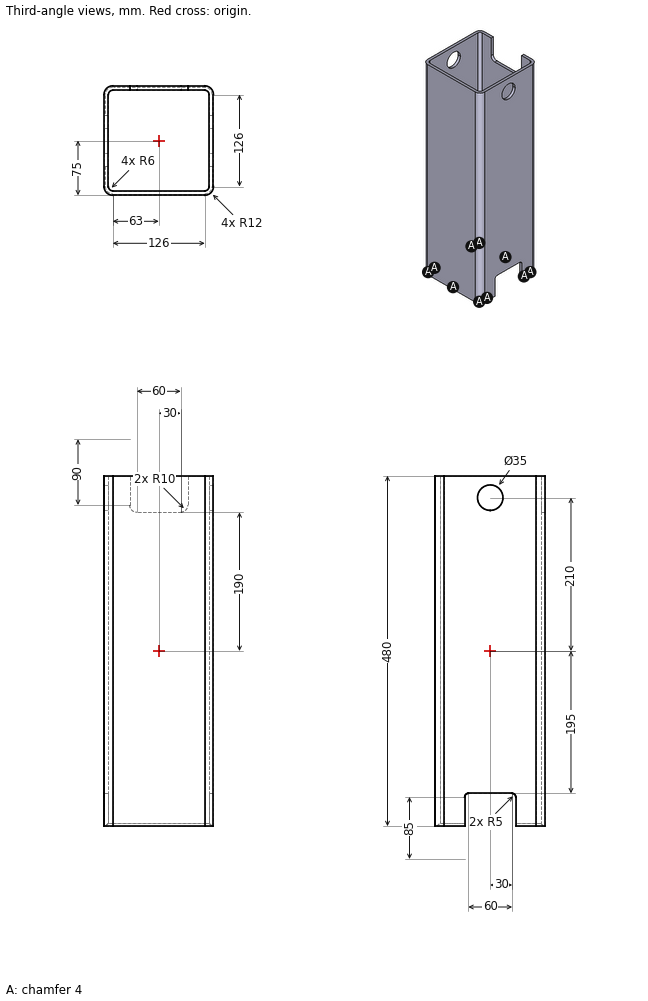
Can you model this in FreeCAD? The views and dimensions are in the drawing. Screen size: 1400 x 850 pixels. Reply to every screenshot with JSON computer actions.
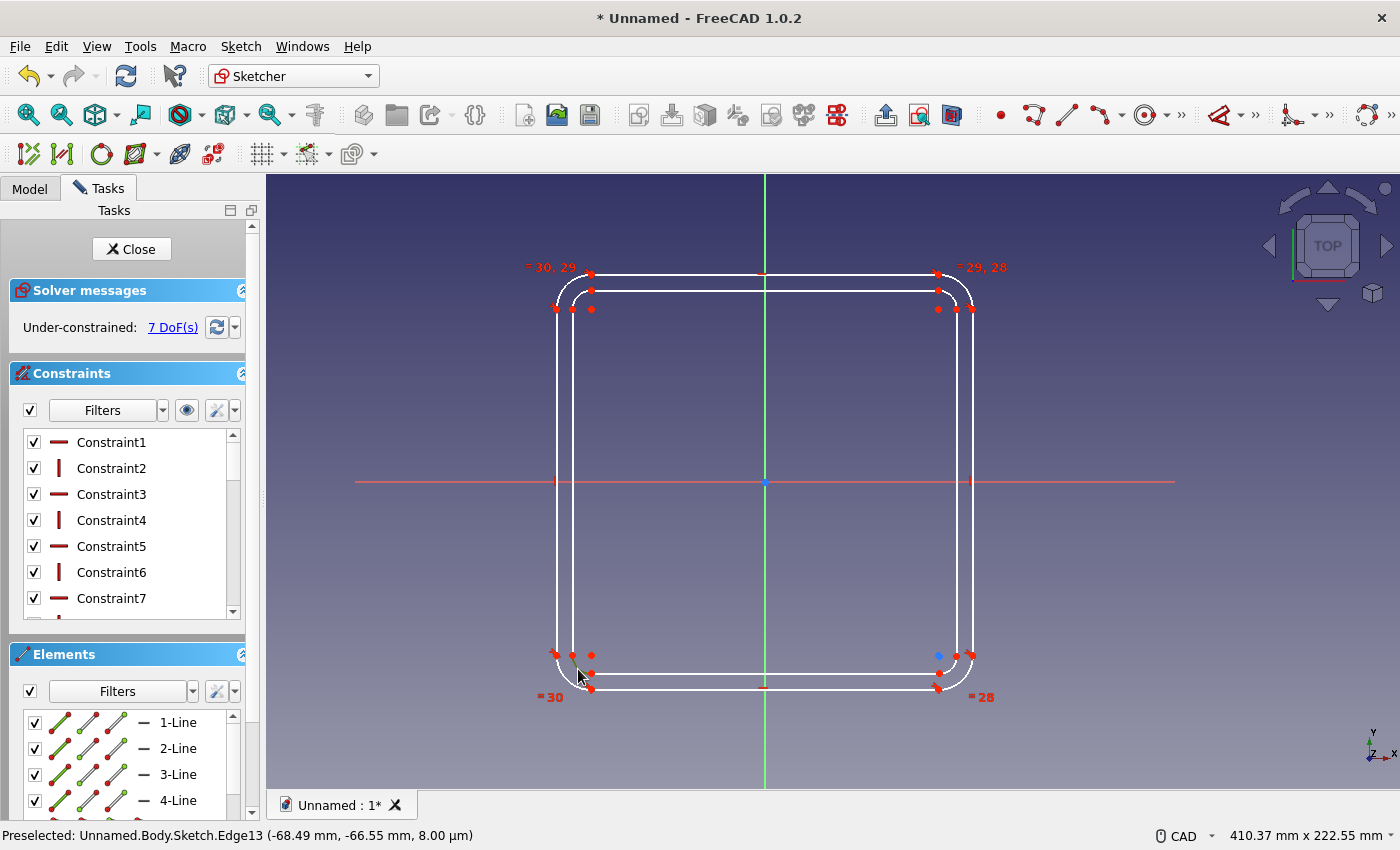
{"action": "left_click", "coordinate": [952, 669]}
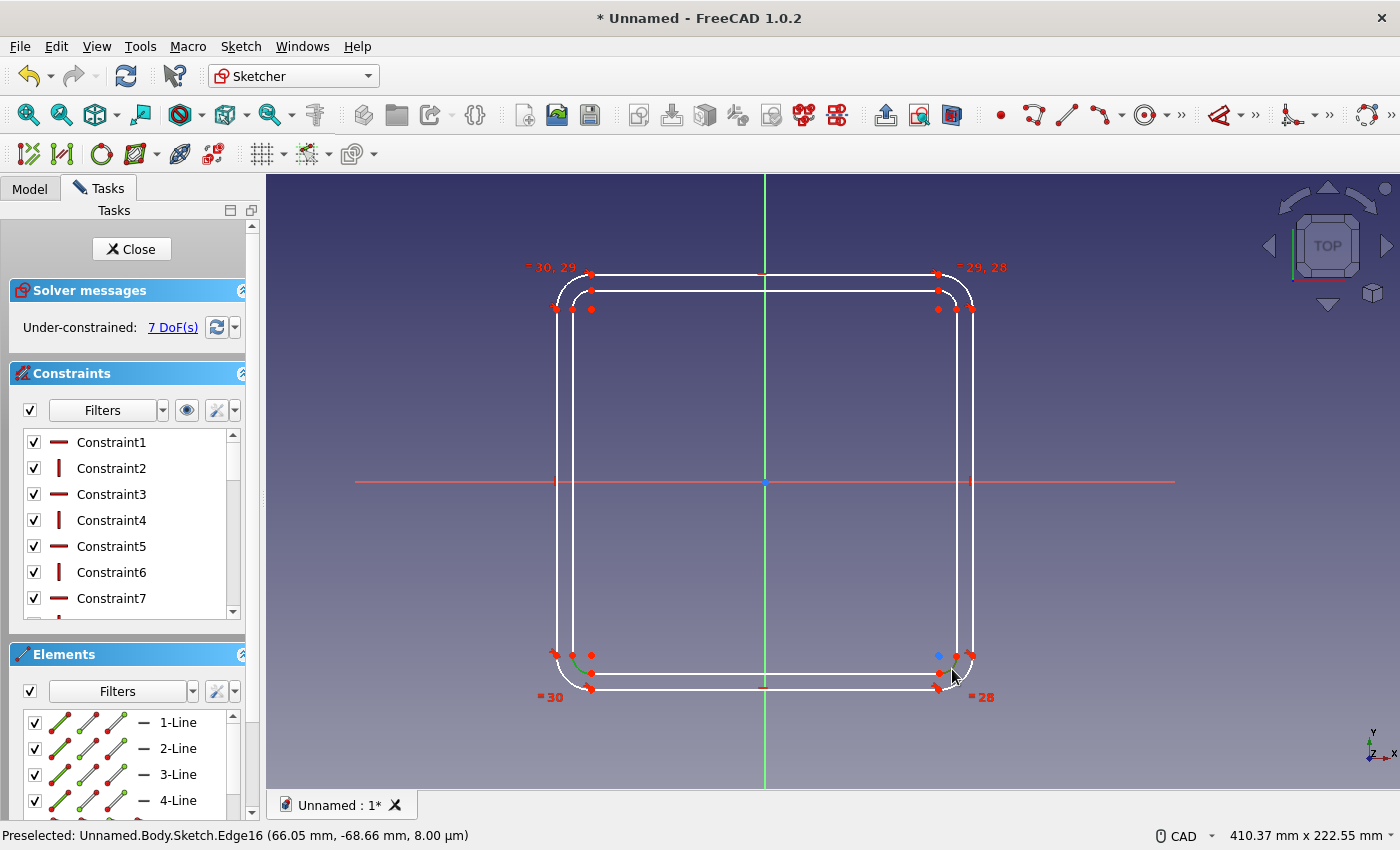
{"action": "key", "text": "e"}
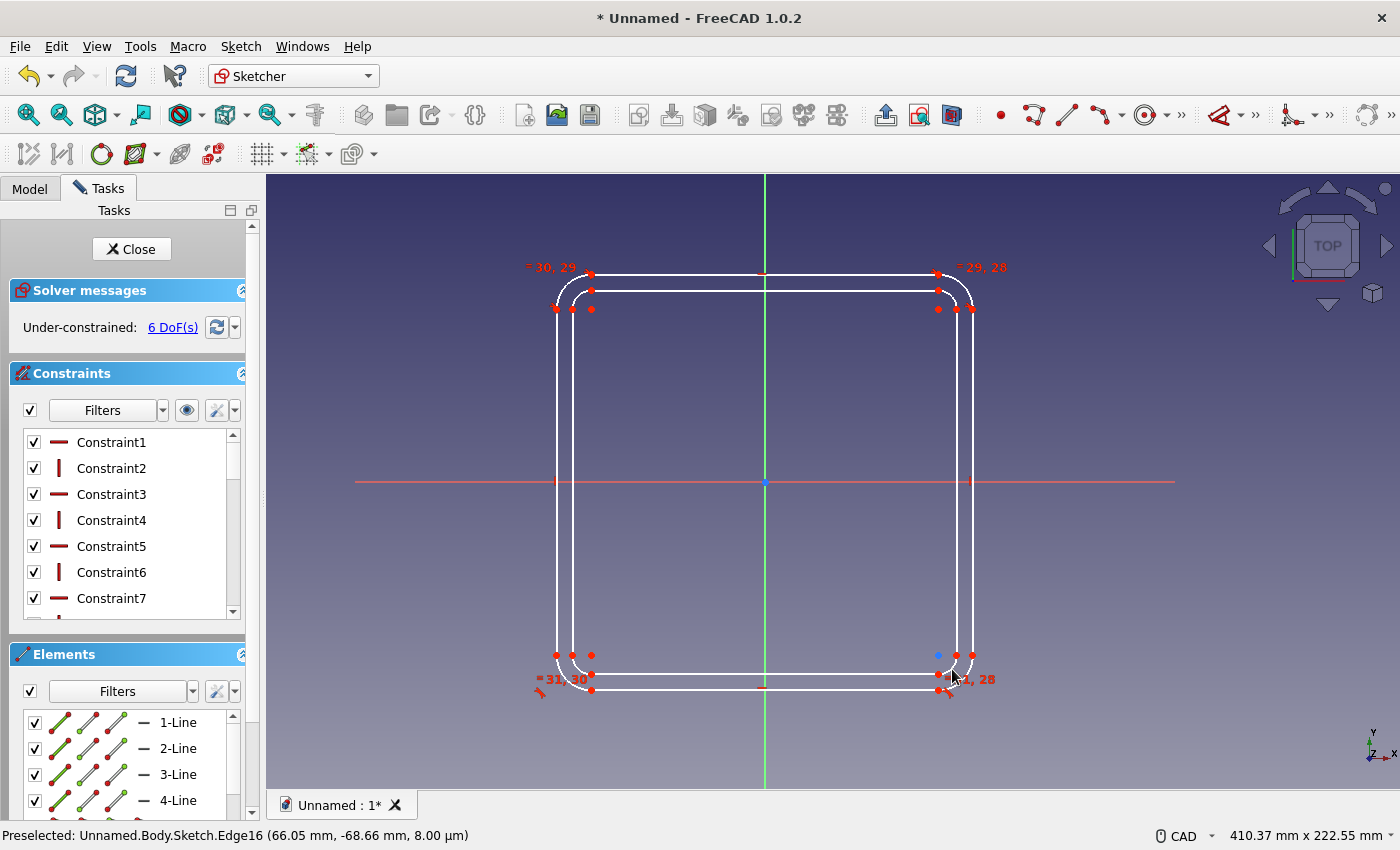
{"action": "left_click", "coordinate": [971, 667]}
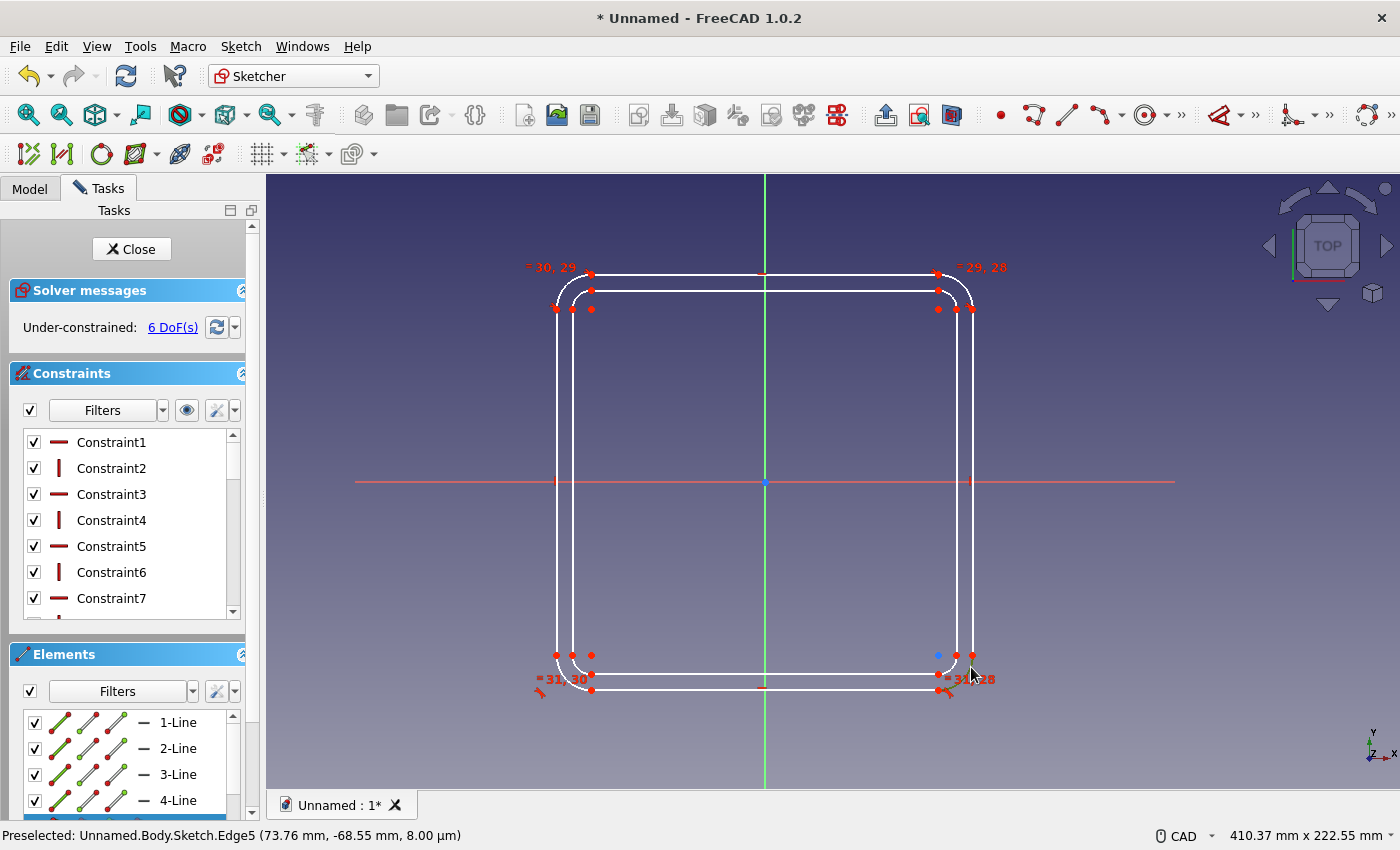
{"action": "key", "text": "k r"}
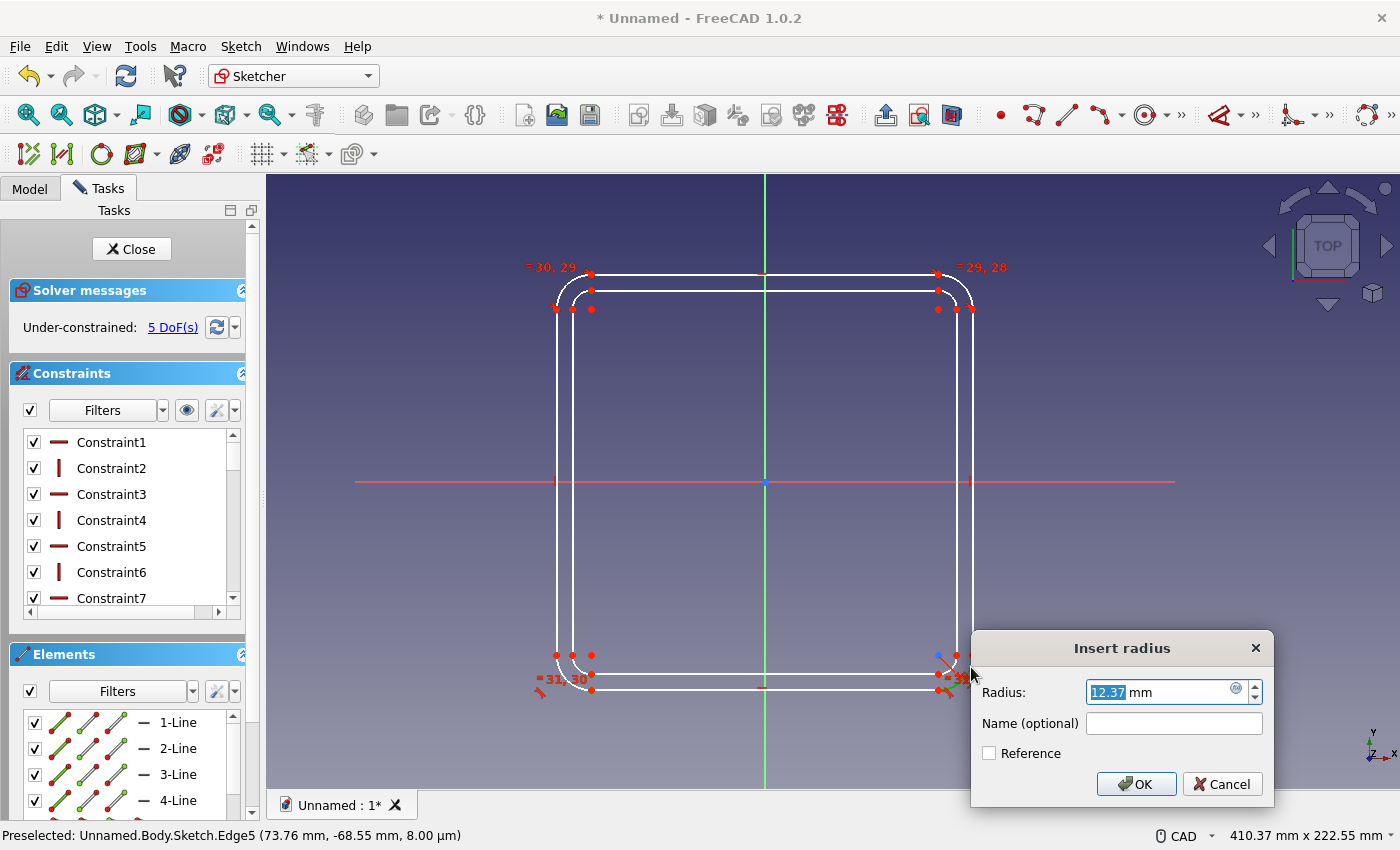
{"action": "type", "text": "12"}
{"action": "key", "text": "Return"}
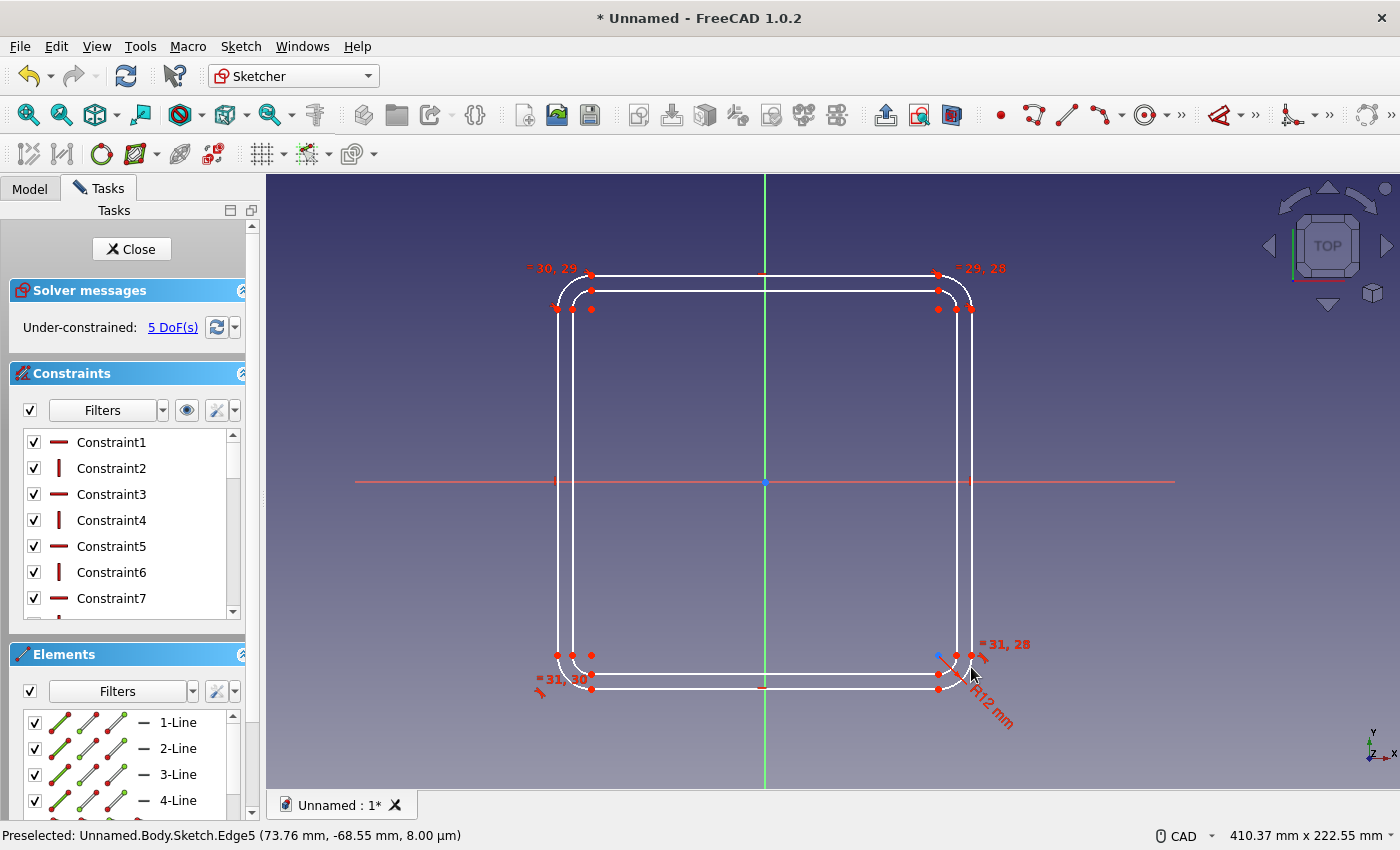
{"action": "scroll", "coordinate": [578, 669], "scroll_direction": "up", "scroll_amount": 5}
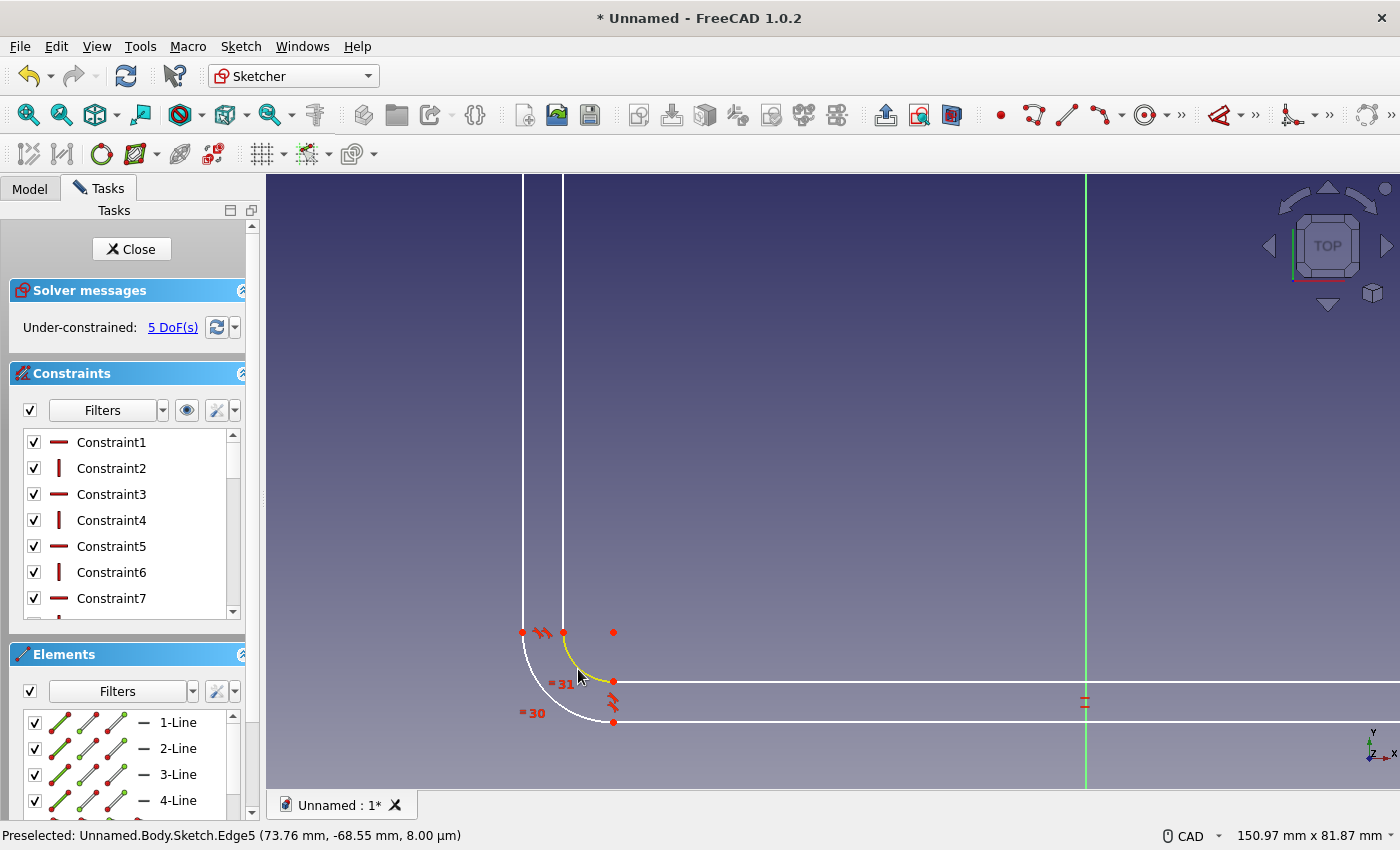
{"action": "left_click", "coordinate": [578, 667]}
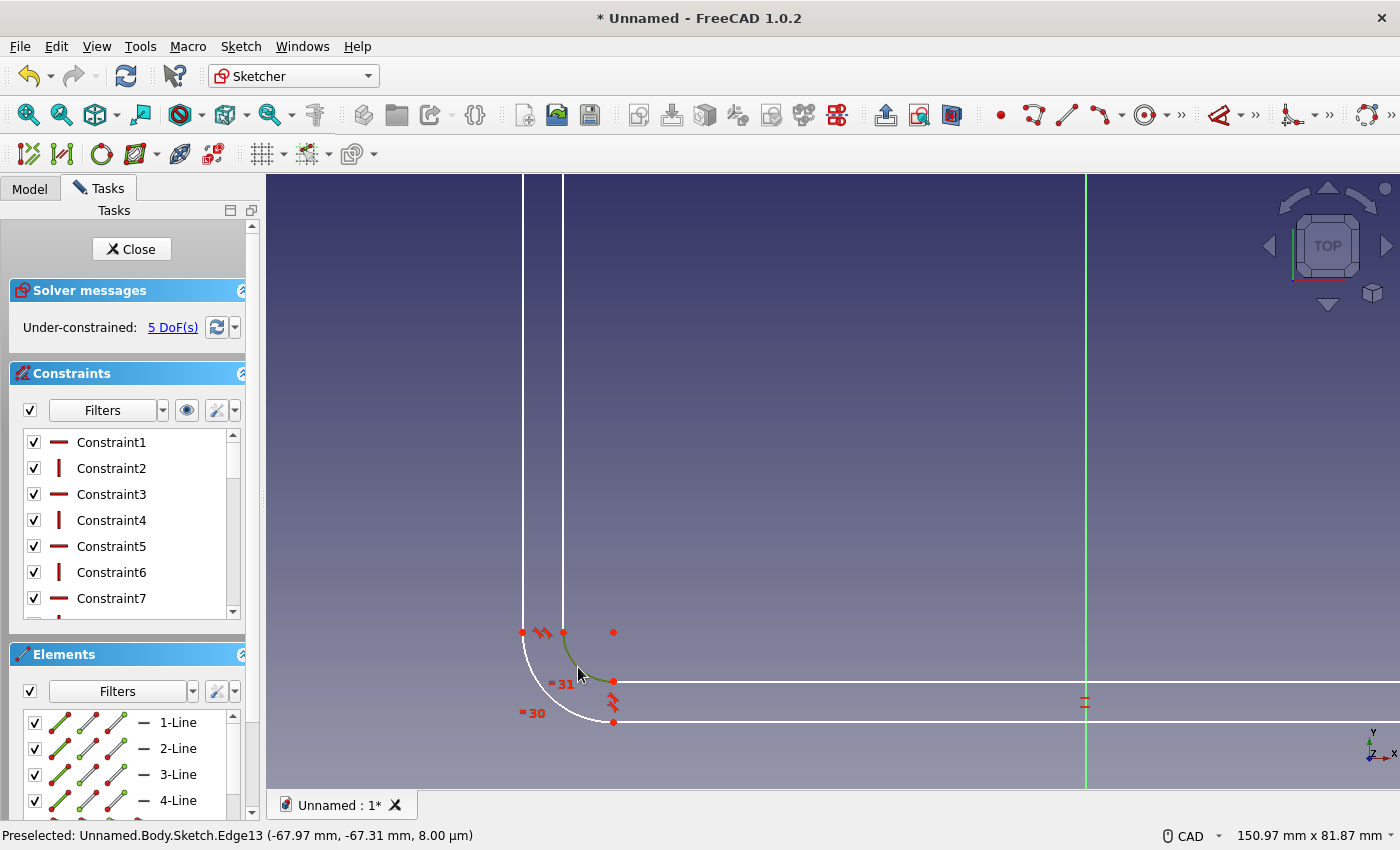
{"action": "key", "text": "k r"}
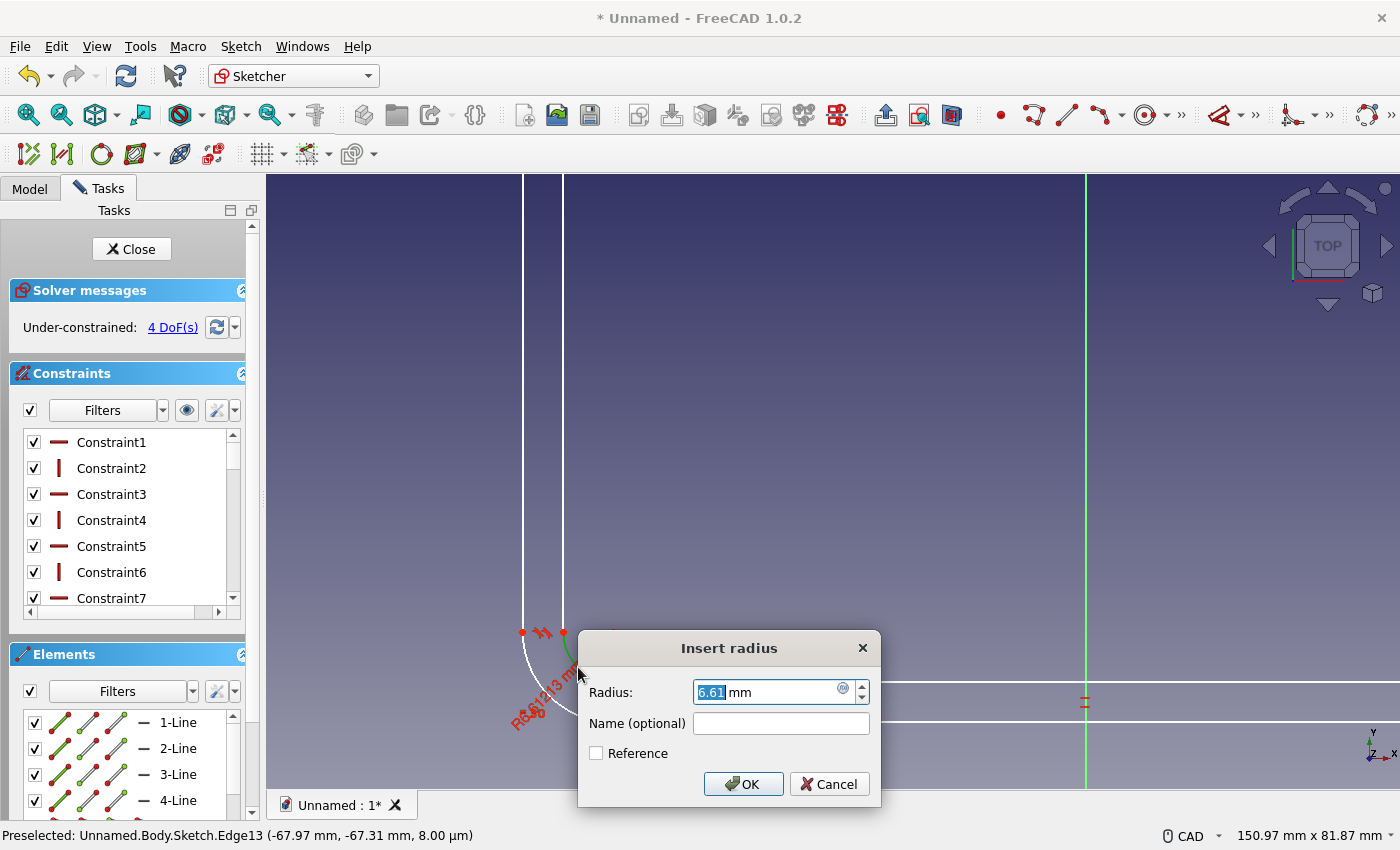
{"action": "type", "text": "6"}
{"action": "key", "text": "Return"}